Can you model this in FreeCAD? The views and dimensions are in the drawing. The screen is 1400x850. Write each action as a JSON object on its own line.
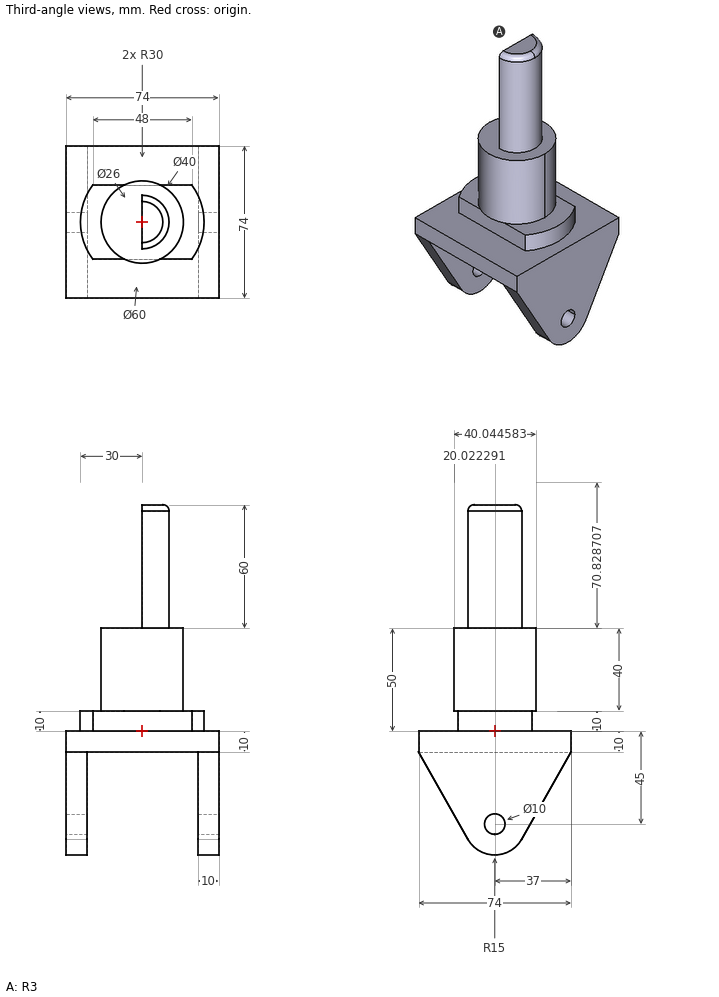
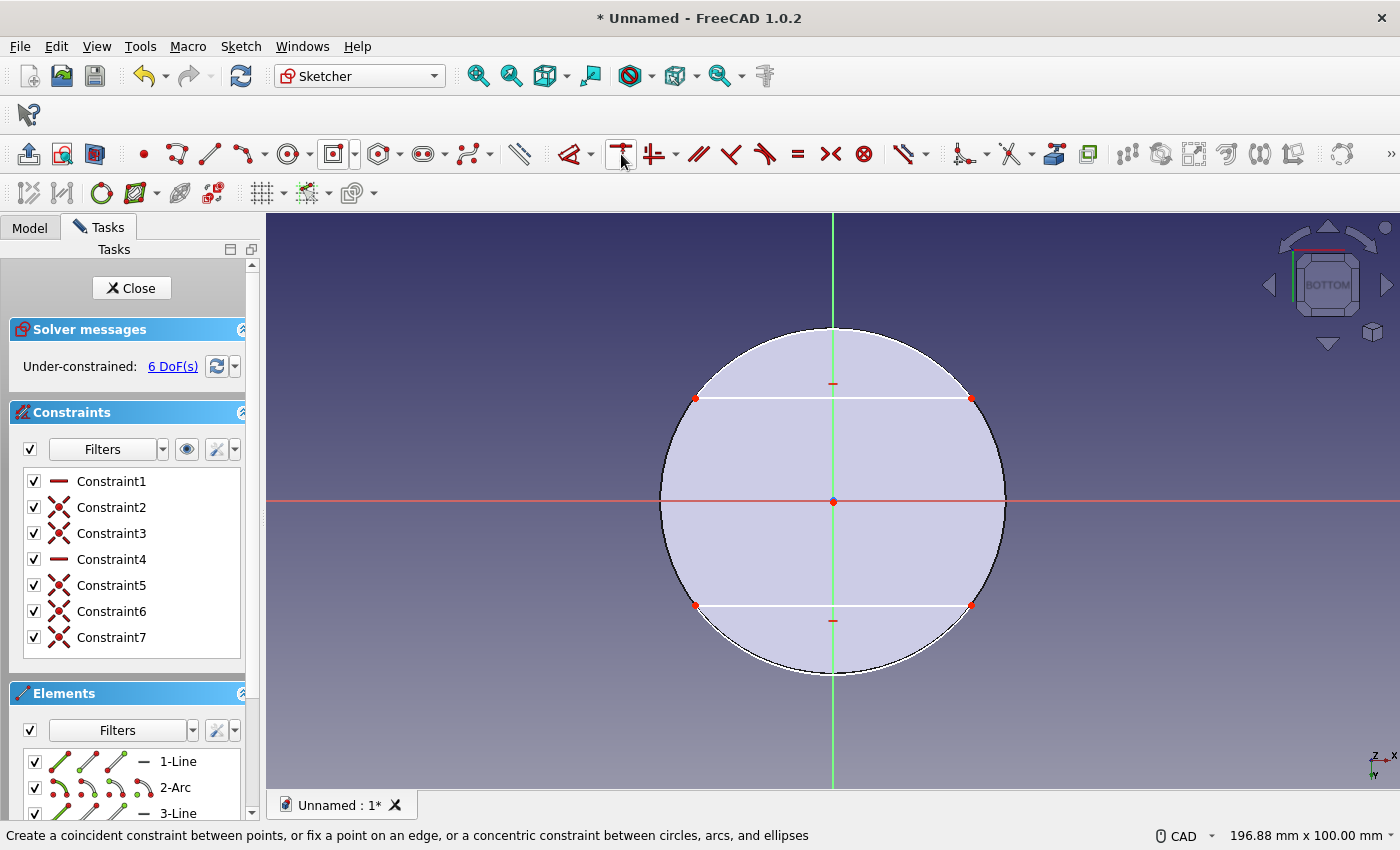
{"action": "left_click_drag", "start_coordinate": [823, 491], "coordinate": [843, 512]}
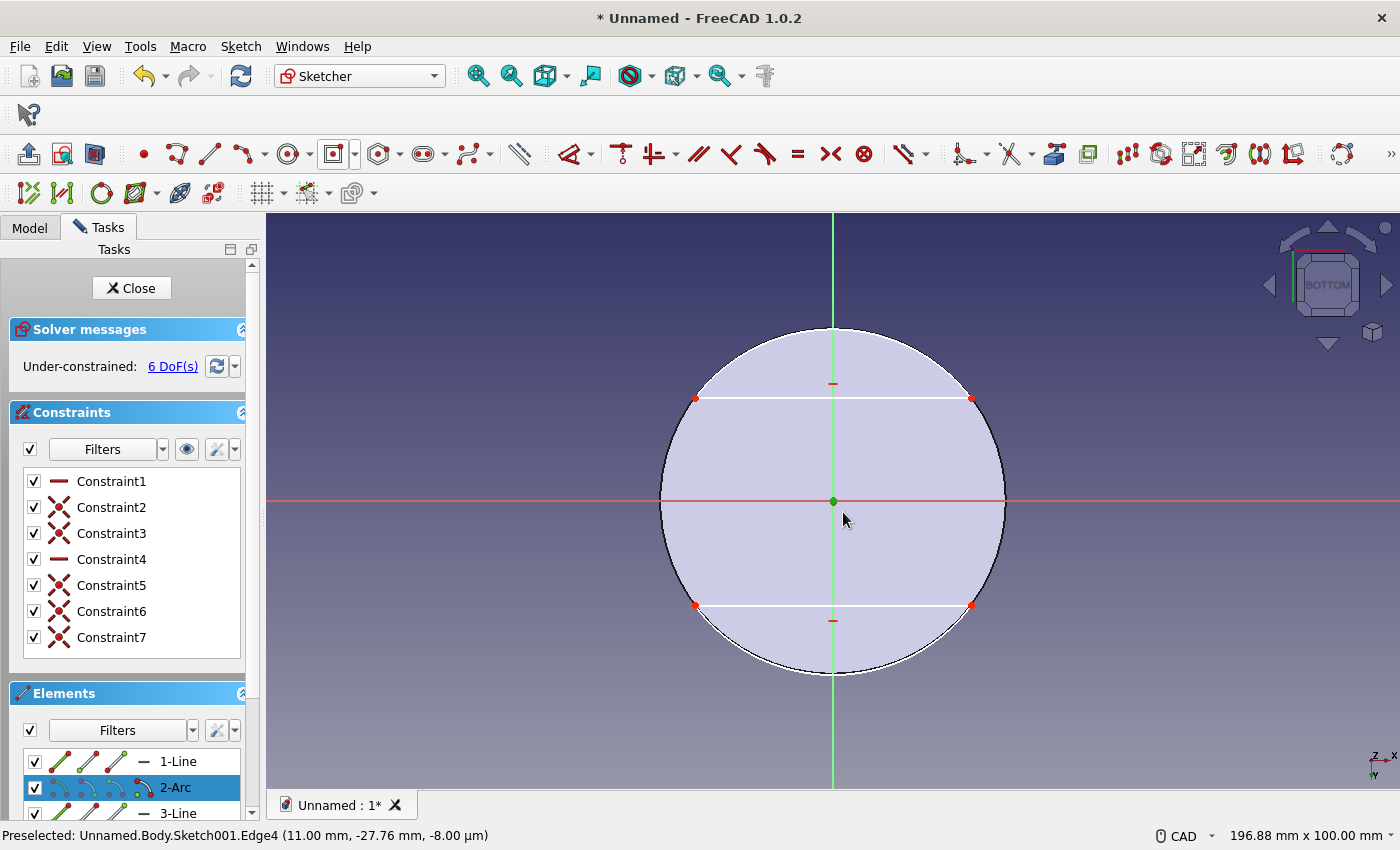
{"action": "left_click", "coordinate": [621, 154]}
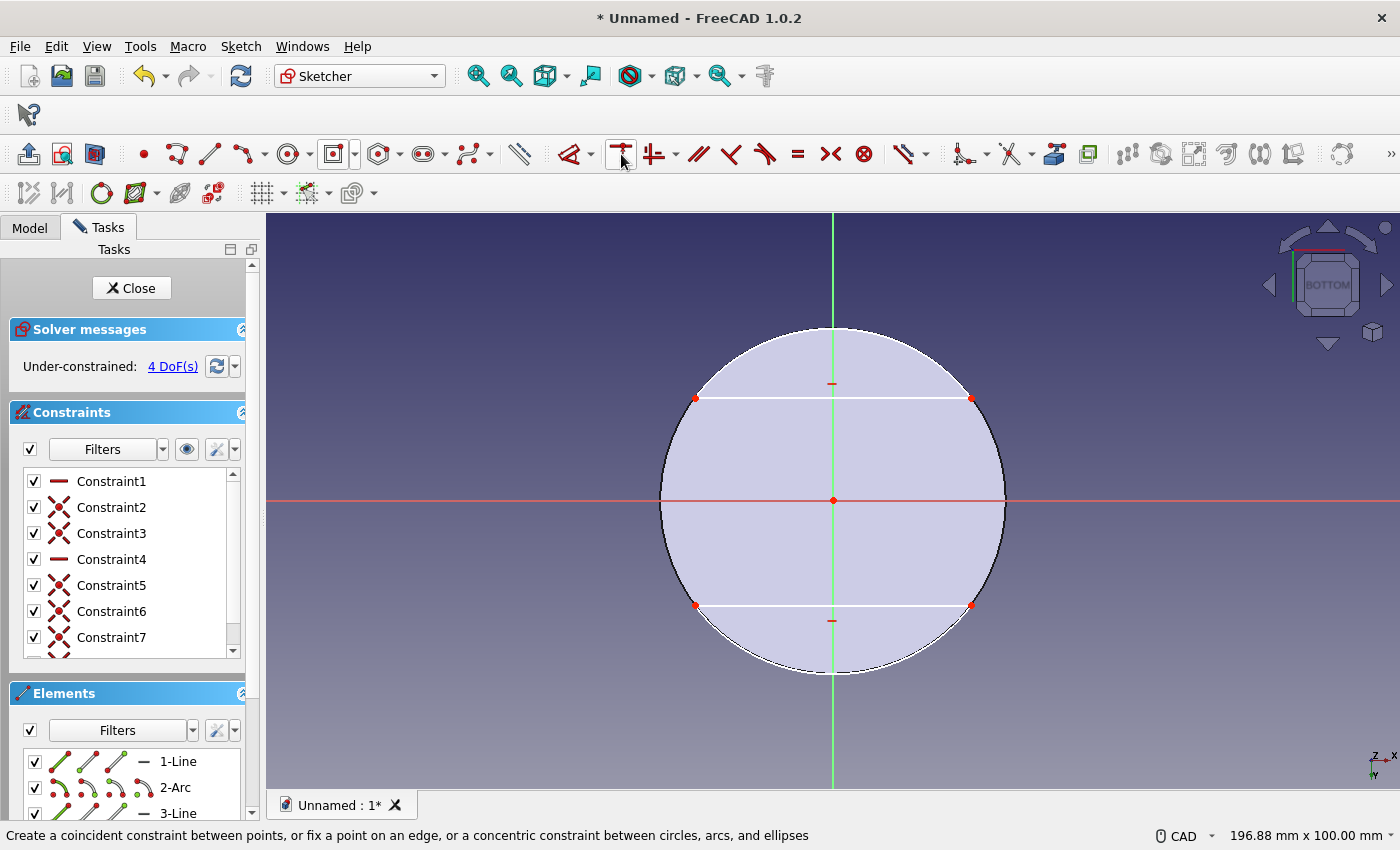
{"action": "left_click", "coordinate": [771, 663]}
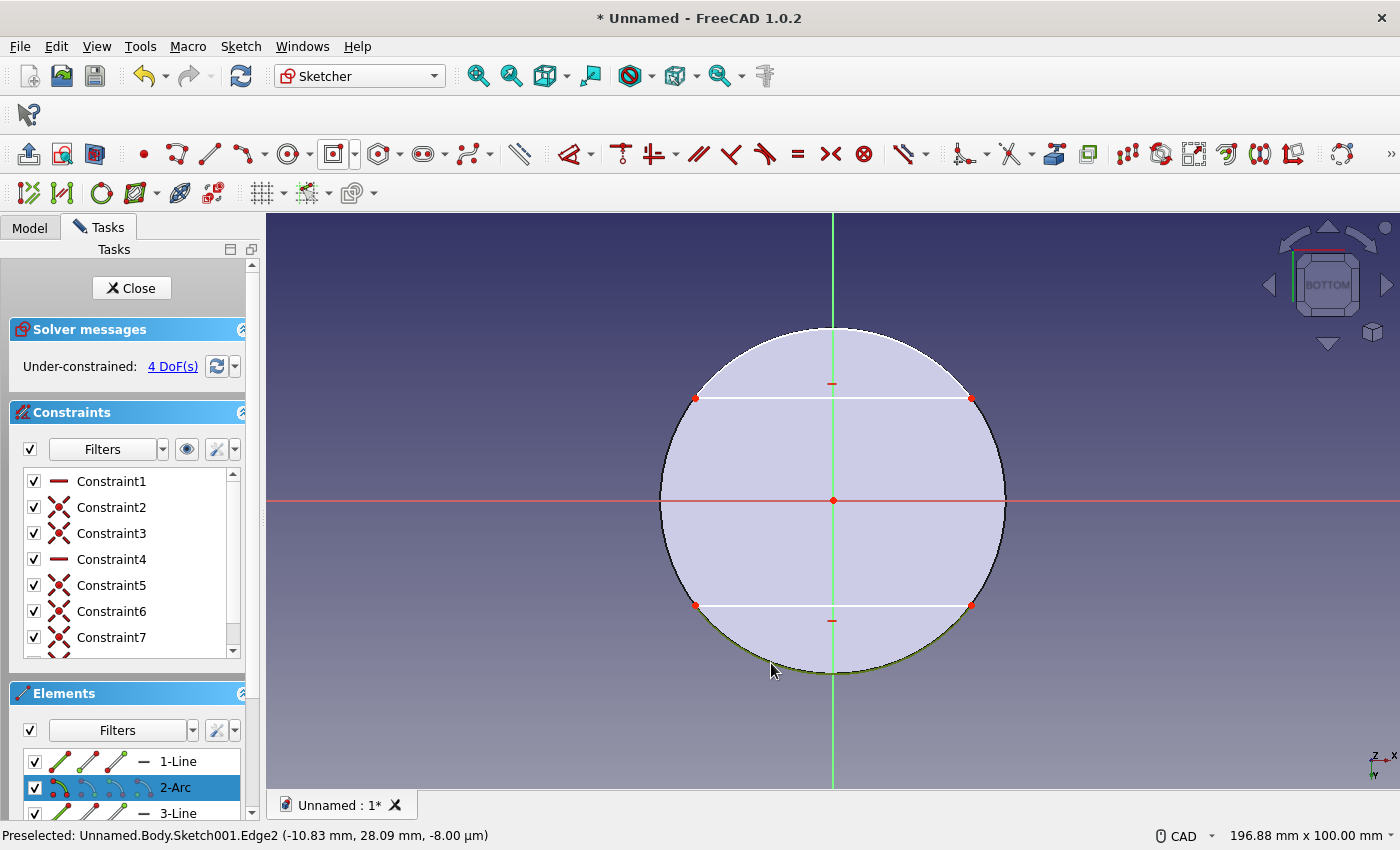
{"action": "left_click", "coordinate": [896, 341]}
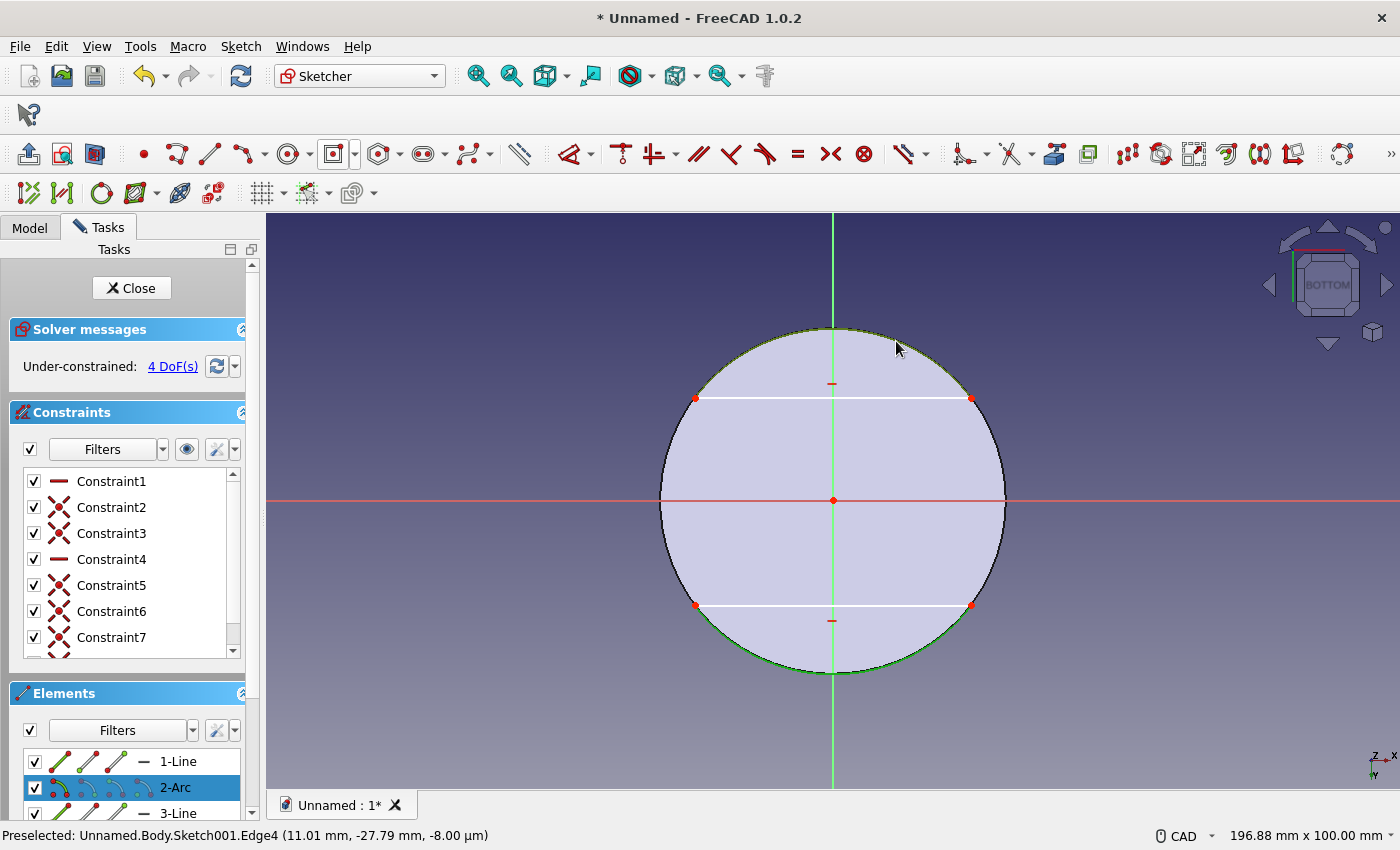
{"action": "key", "text": "e"}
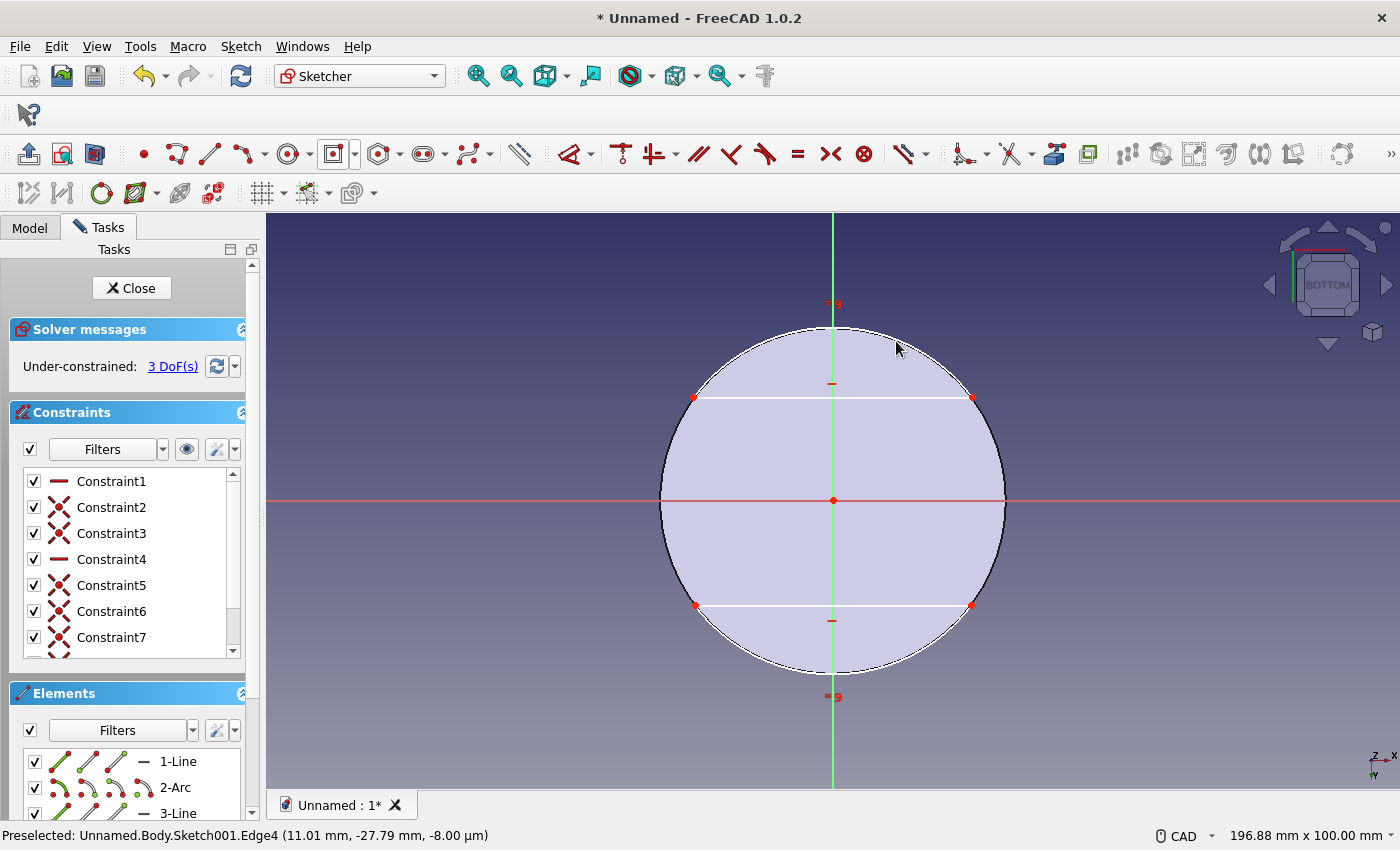
{"action": "left_click", "coordinate": [568, 154]}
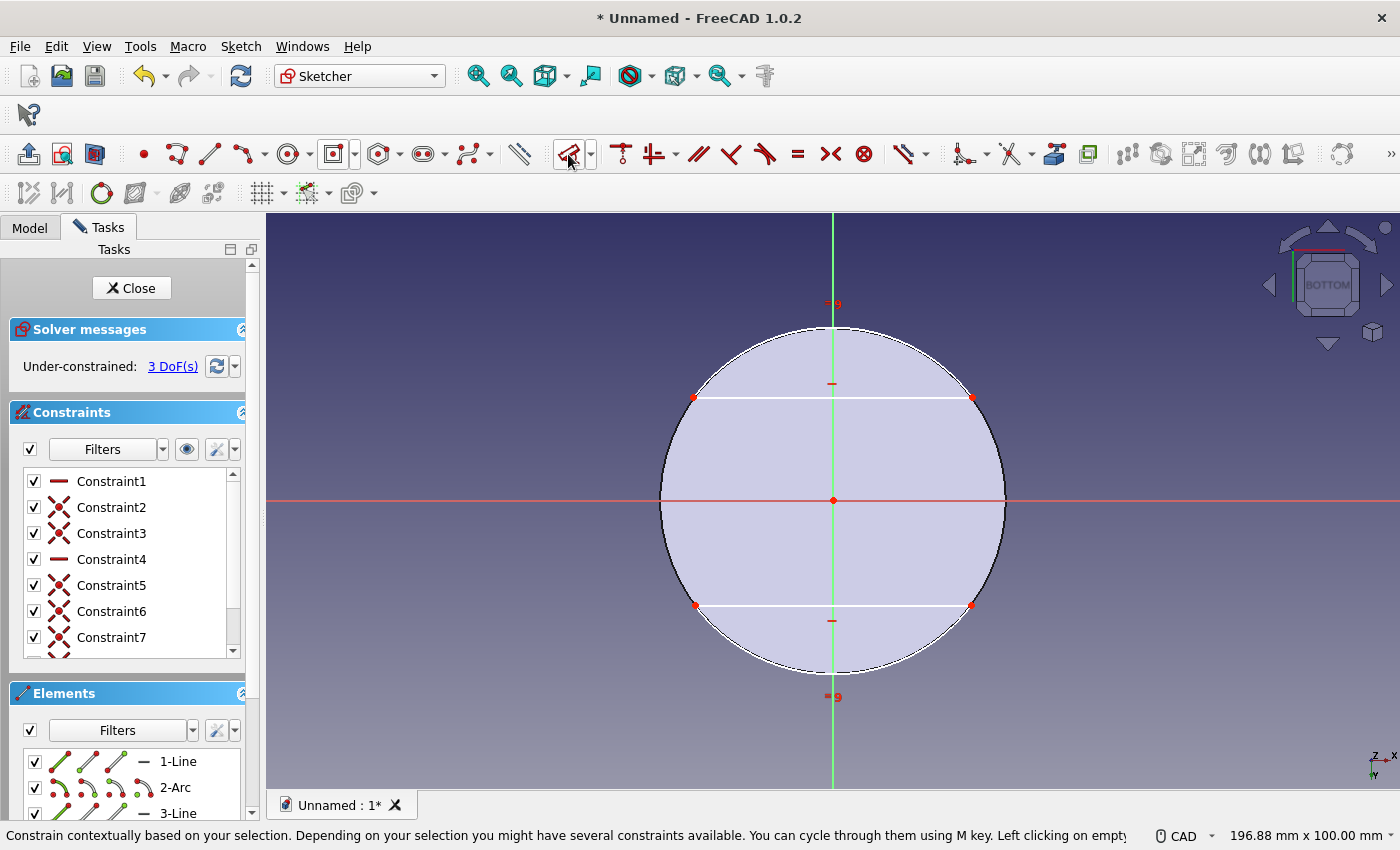
{"action": "left_click", "coordinate": [771, 663]}
{"action": "left_click", "coordinate": [760, 693]}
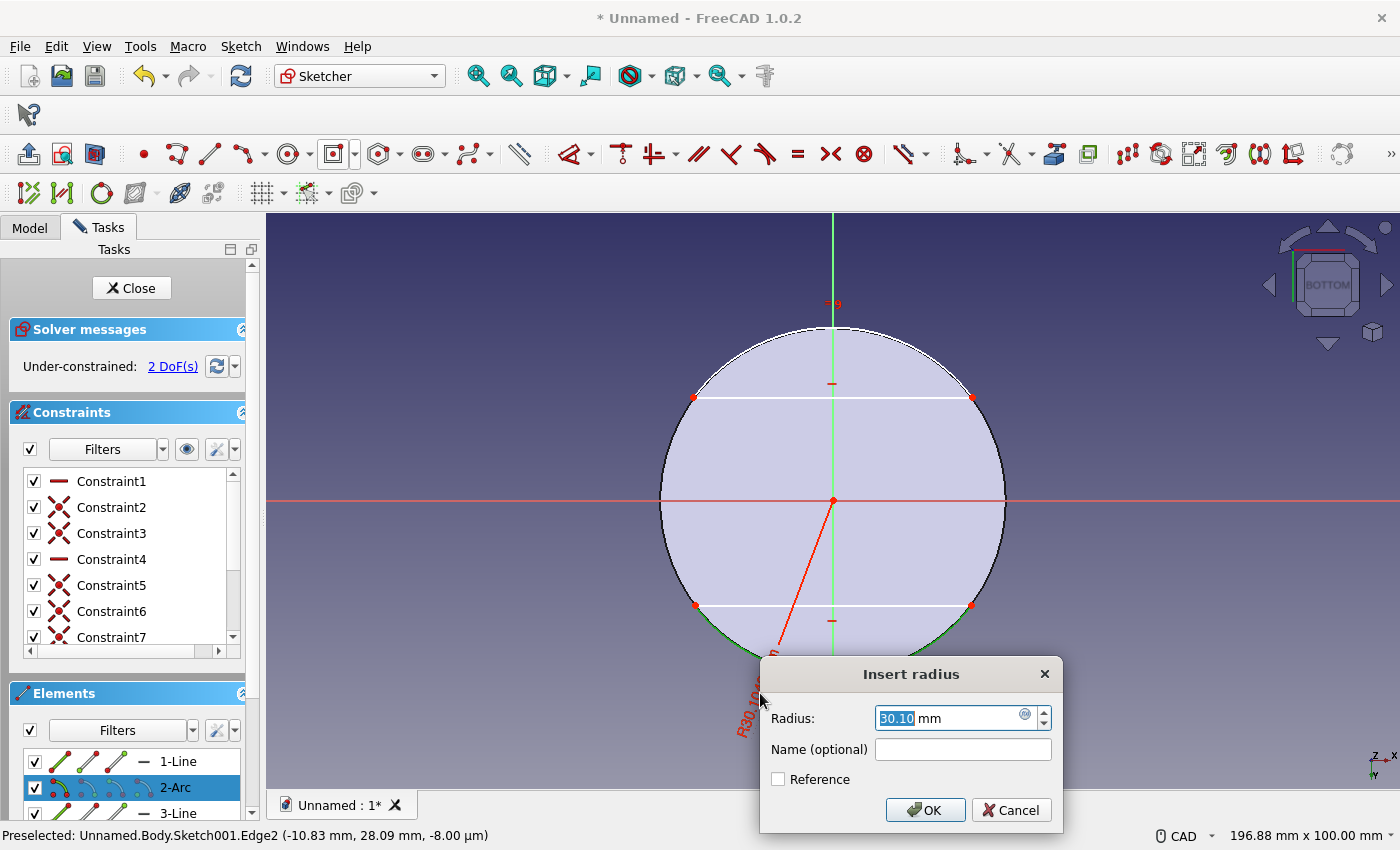
{"action": "type", "text": "30"}
{"action": "key", "text": "Return"}